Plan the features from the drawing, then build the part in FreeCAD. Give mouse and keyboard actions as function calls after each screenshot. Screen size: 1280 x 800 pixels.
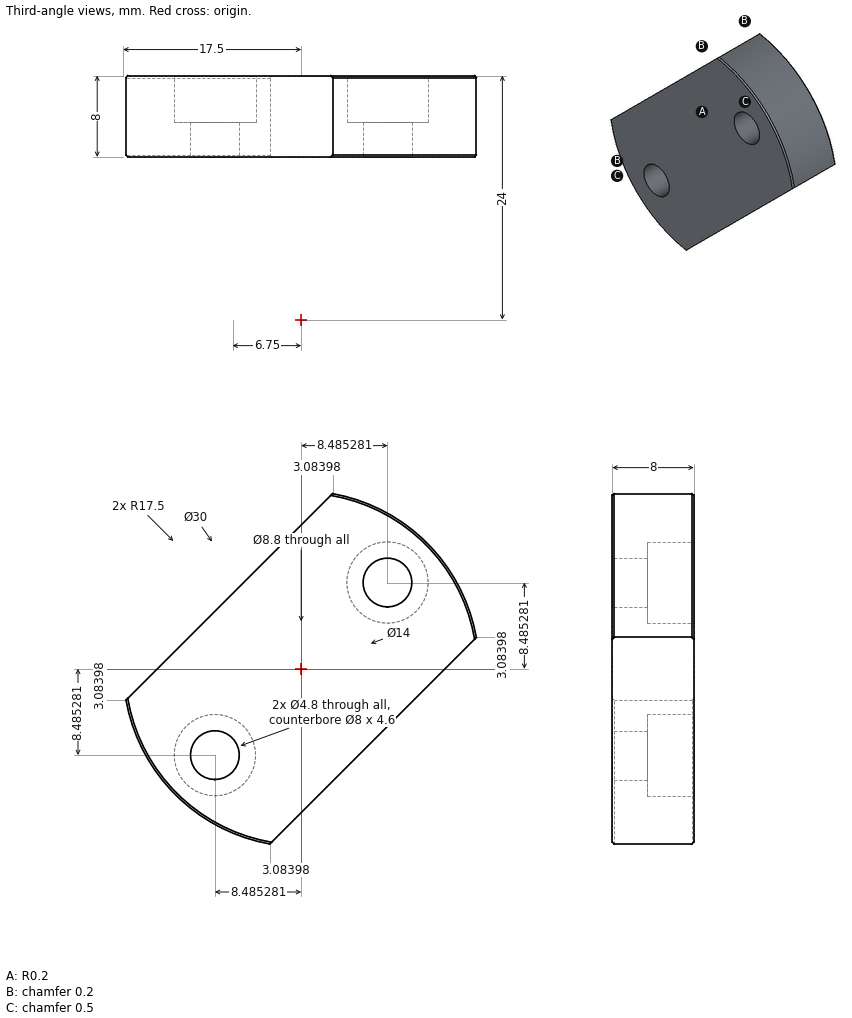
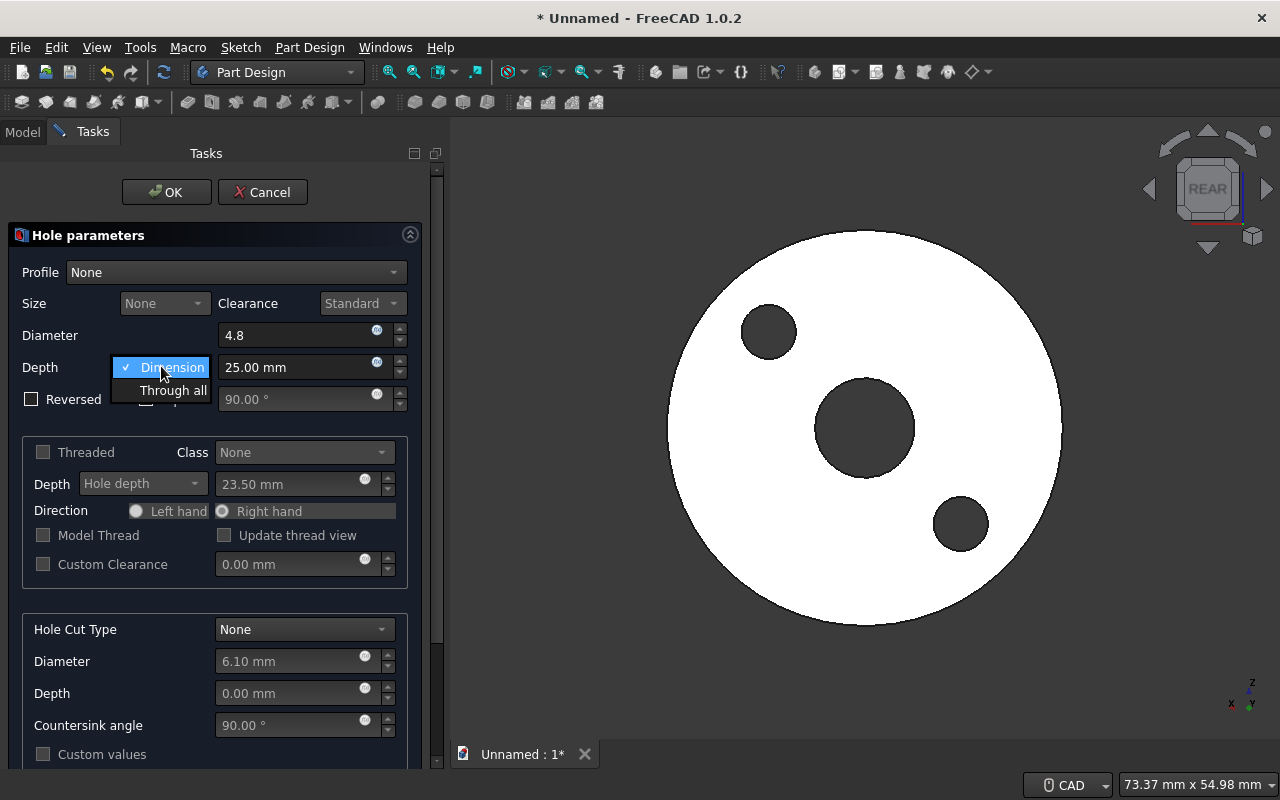
click(160, 390)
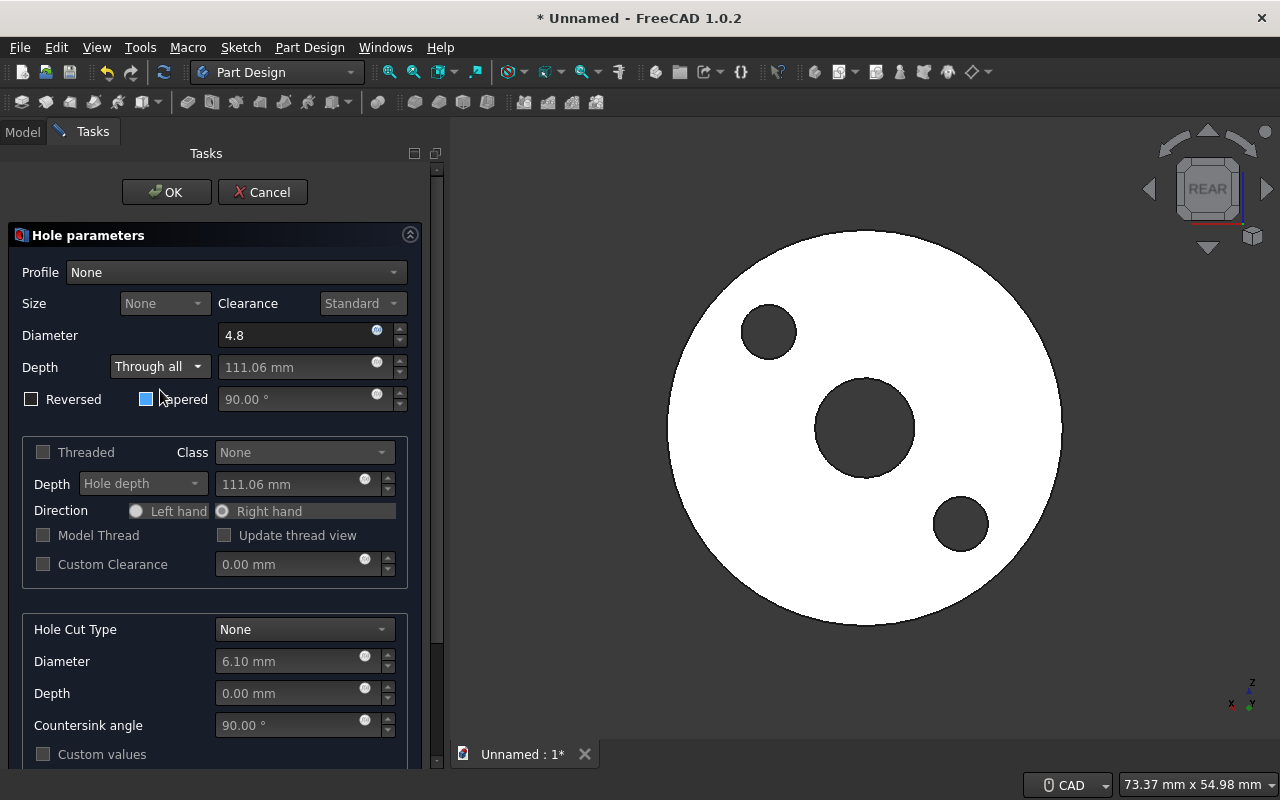
click(306, 630)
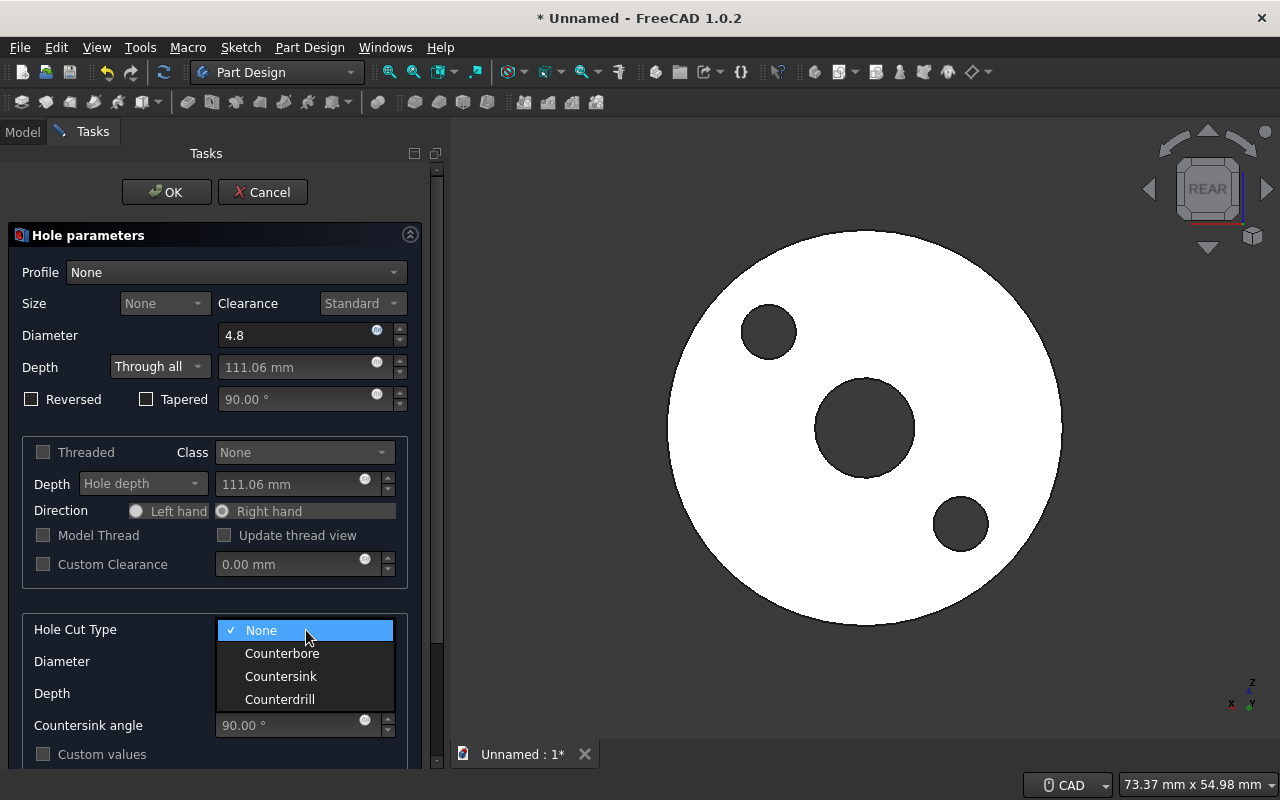
click(304, 654)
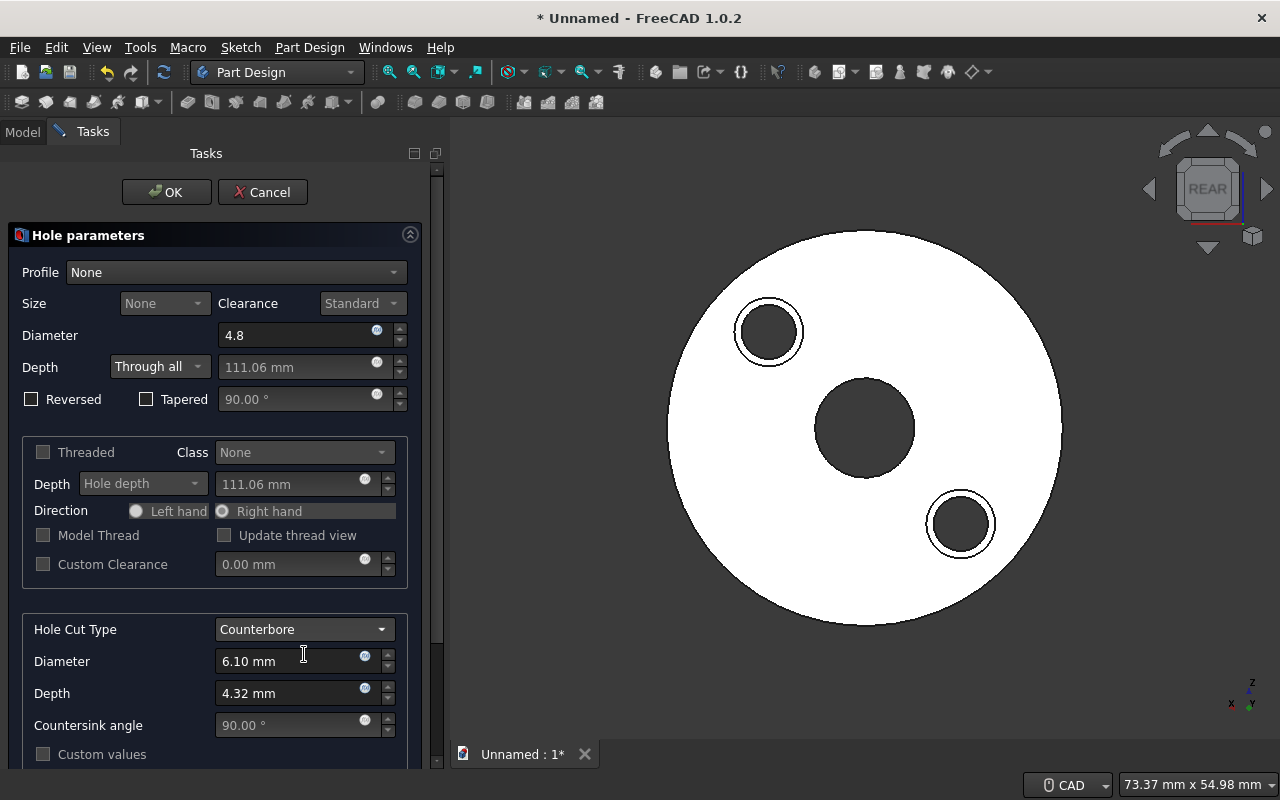
triple_click(298, 661)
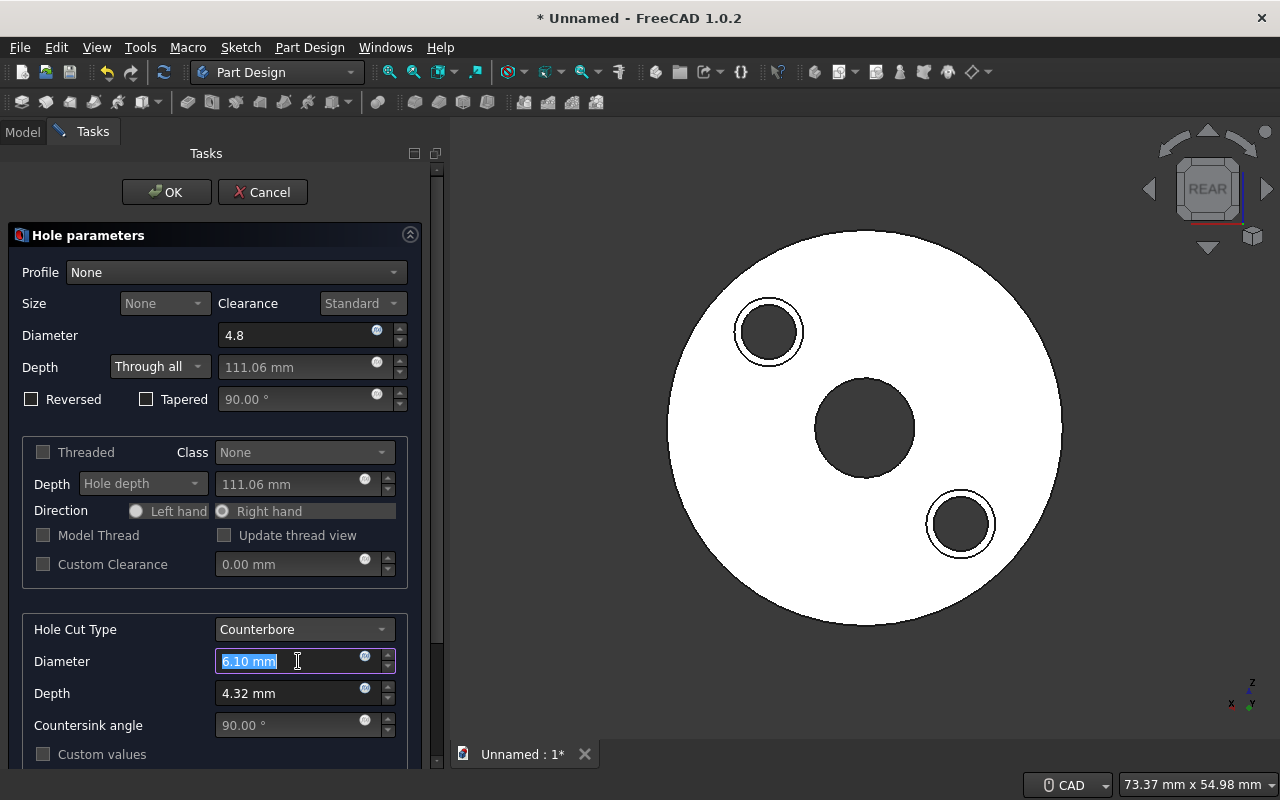
text(8)
key(Tab)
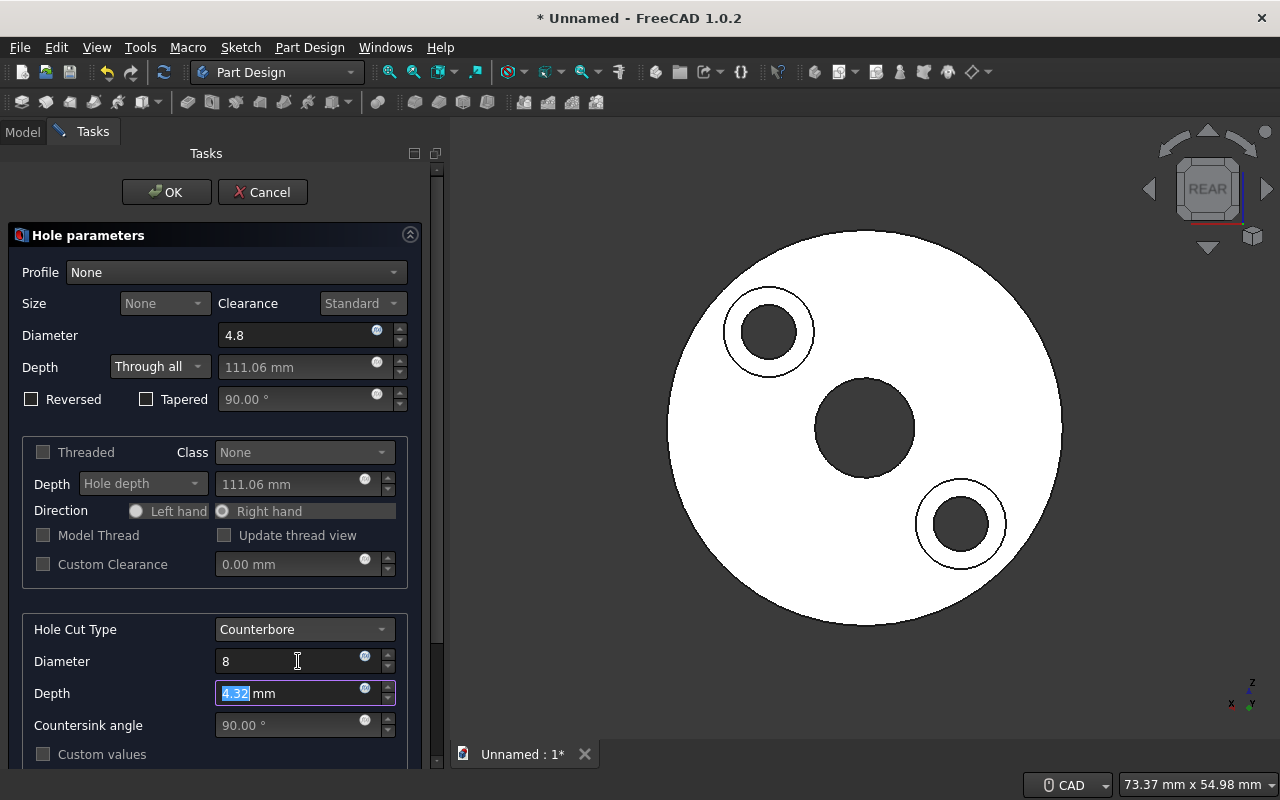
text(4.6)
key(Tab)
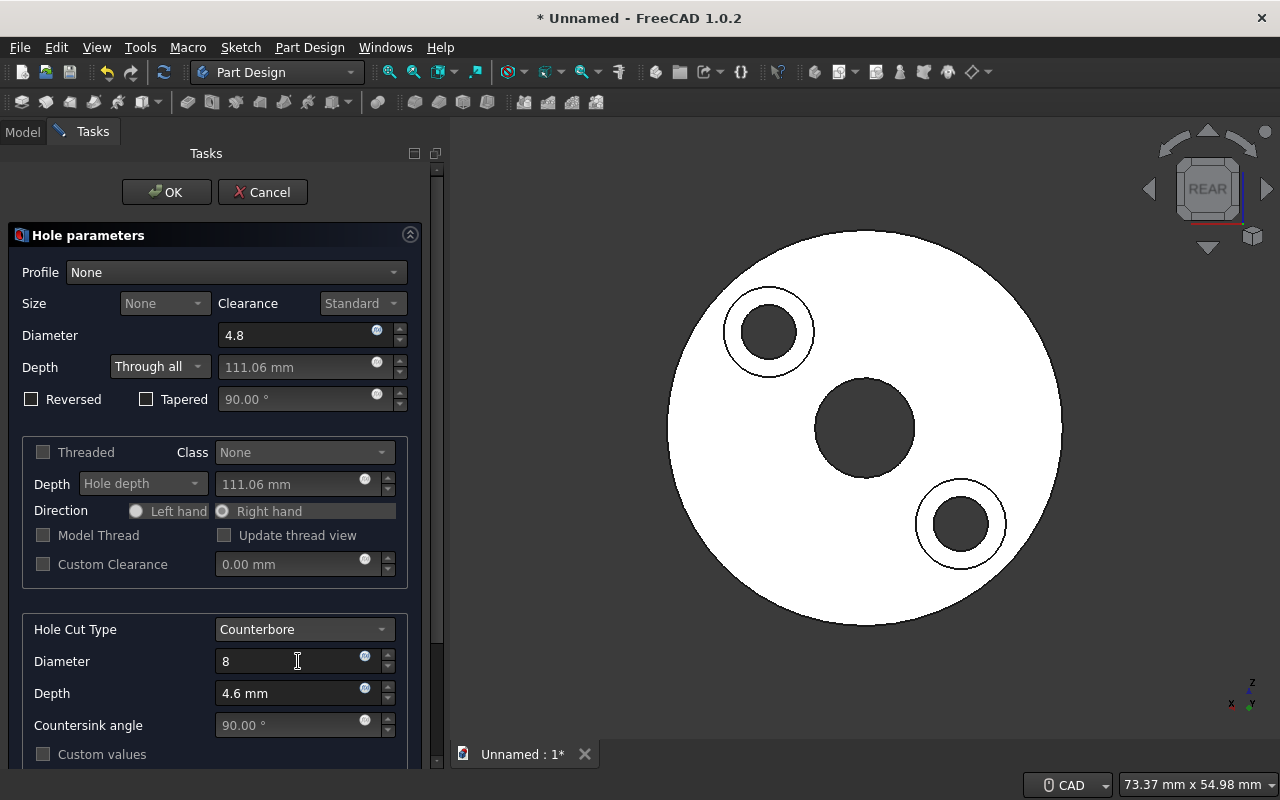
click(167, 192)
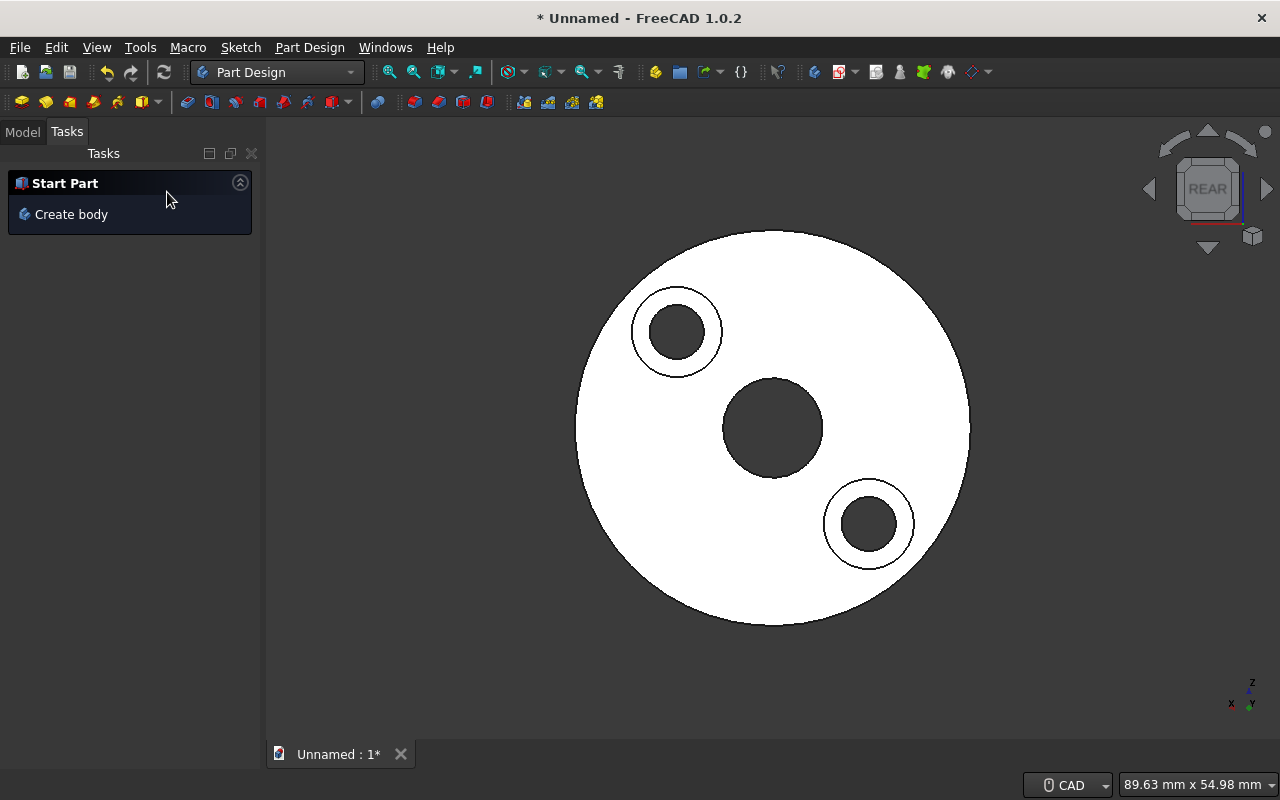
key(0)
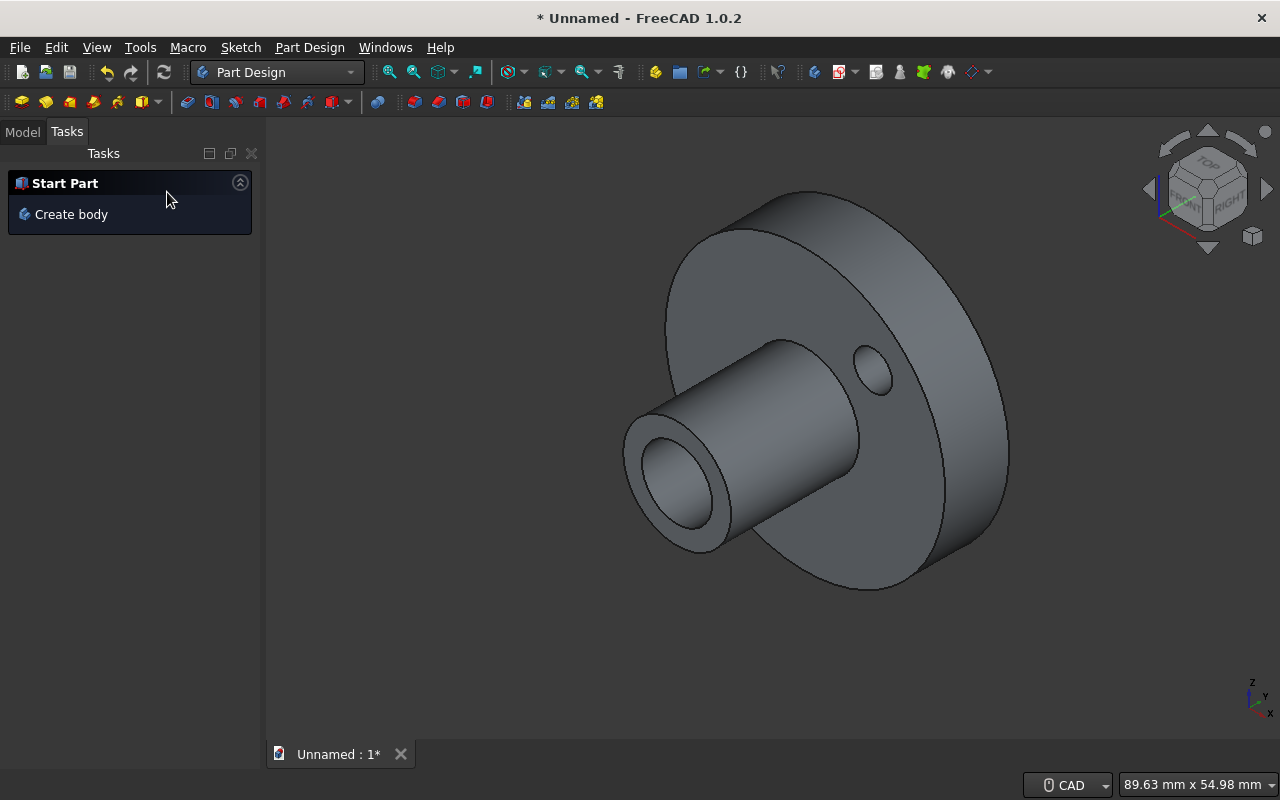
key(2)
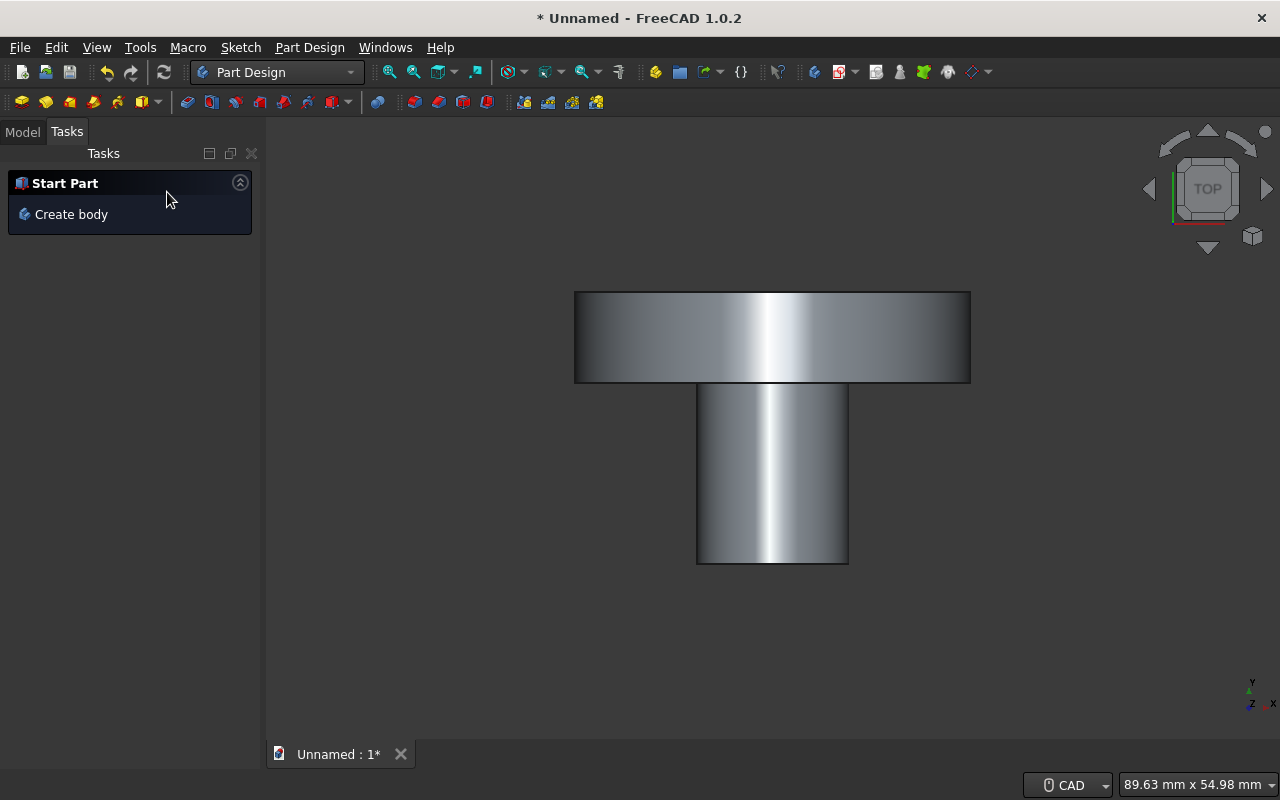
click(390, 72)